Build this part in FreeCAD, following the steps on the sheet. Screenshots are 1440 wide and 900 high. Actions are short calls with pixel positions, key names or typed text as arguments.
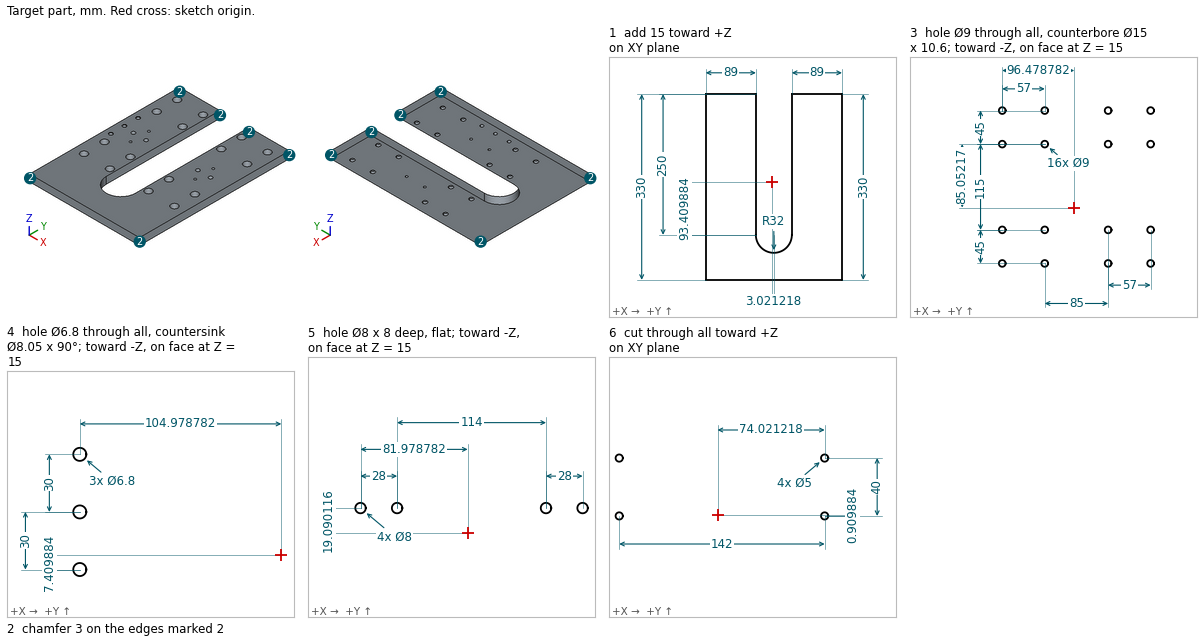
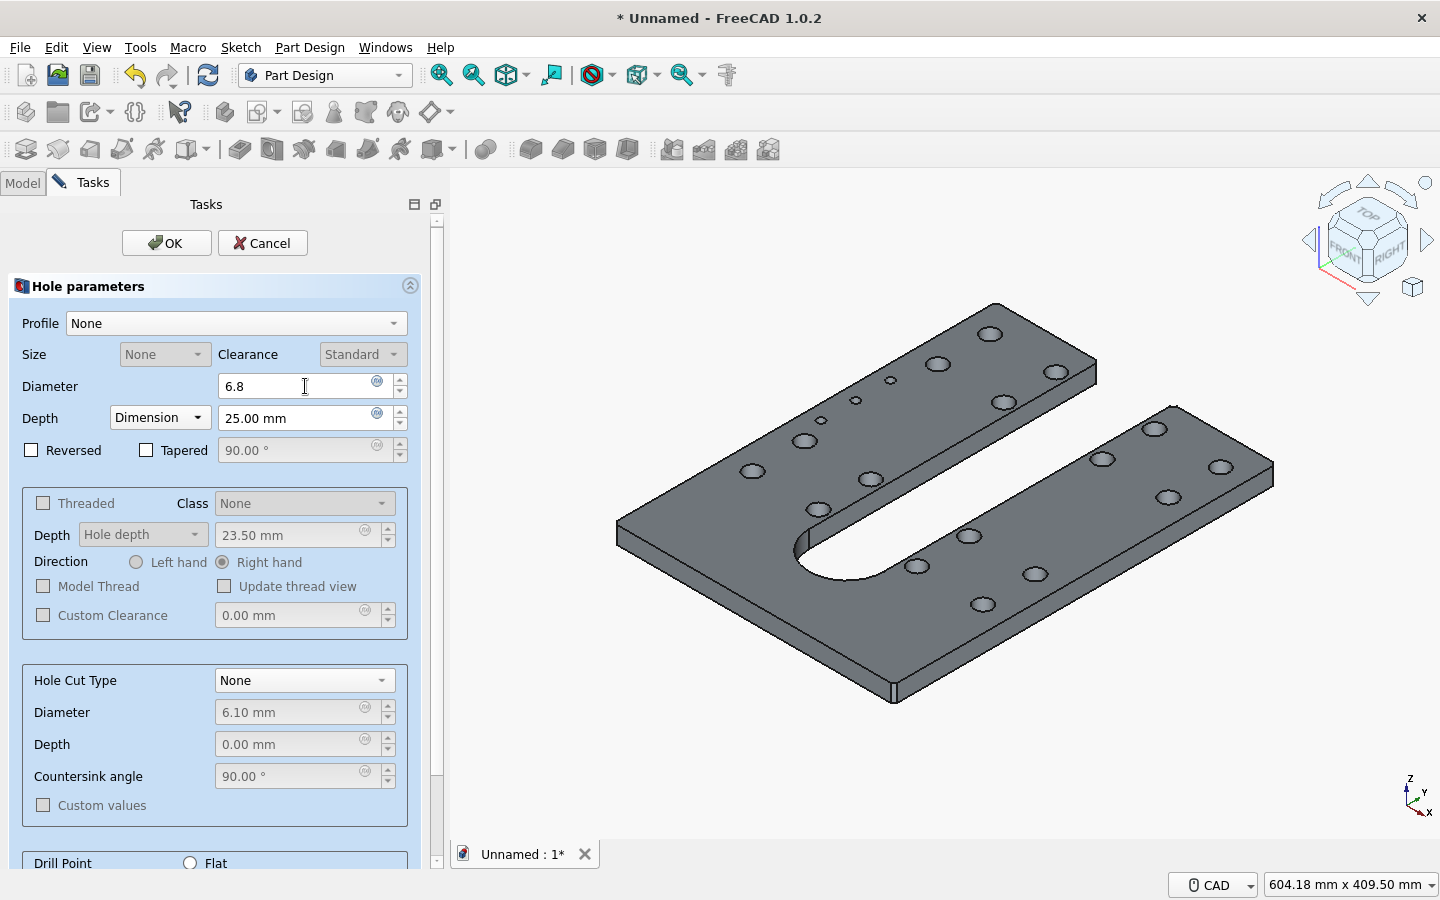
click(161, 418)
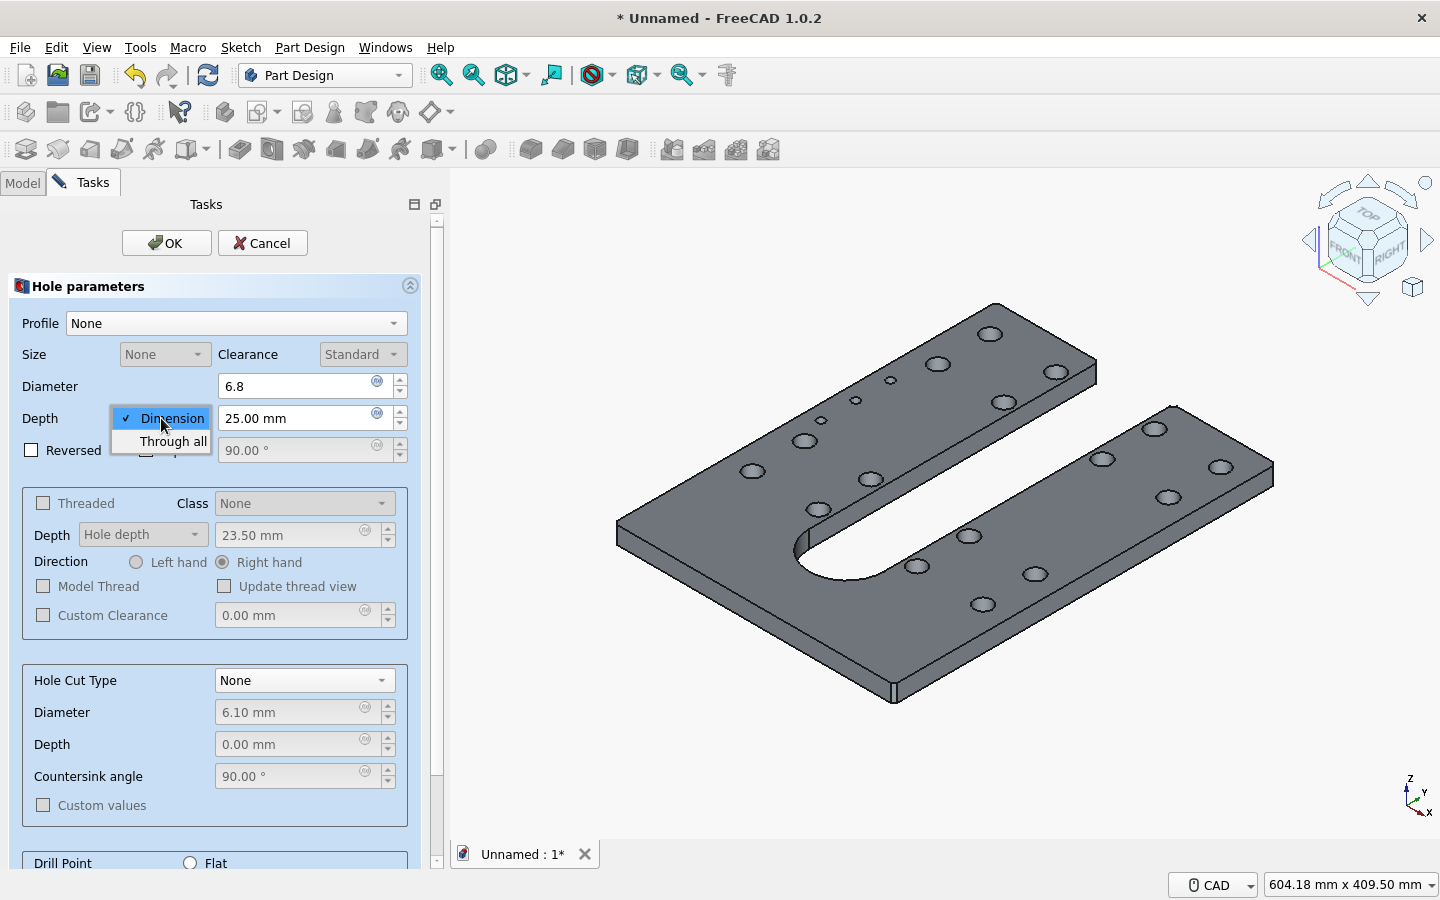
click(160, 442)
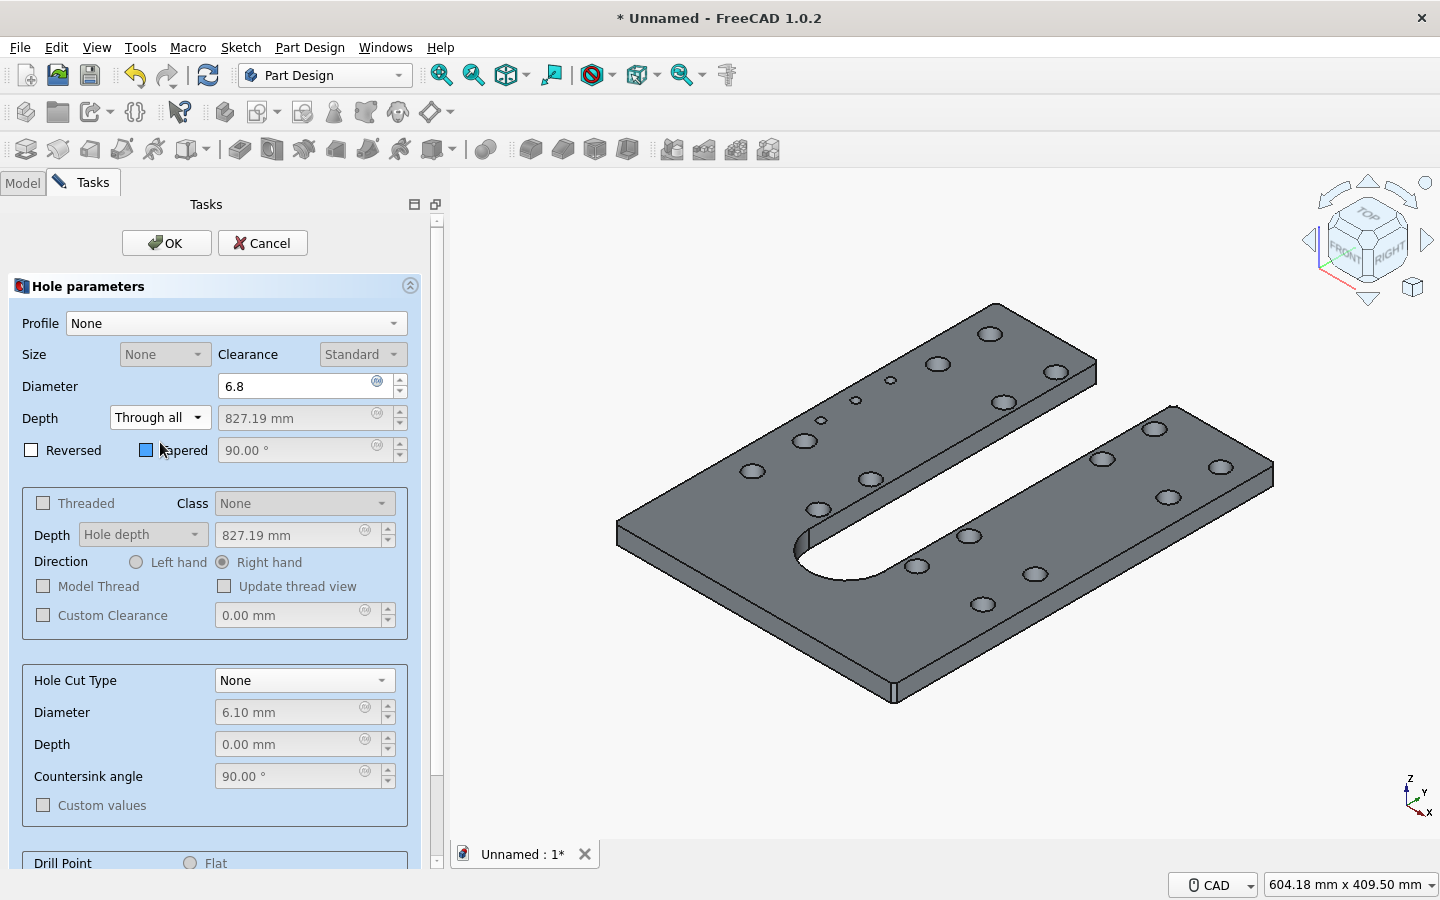
click(306, 680)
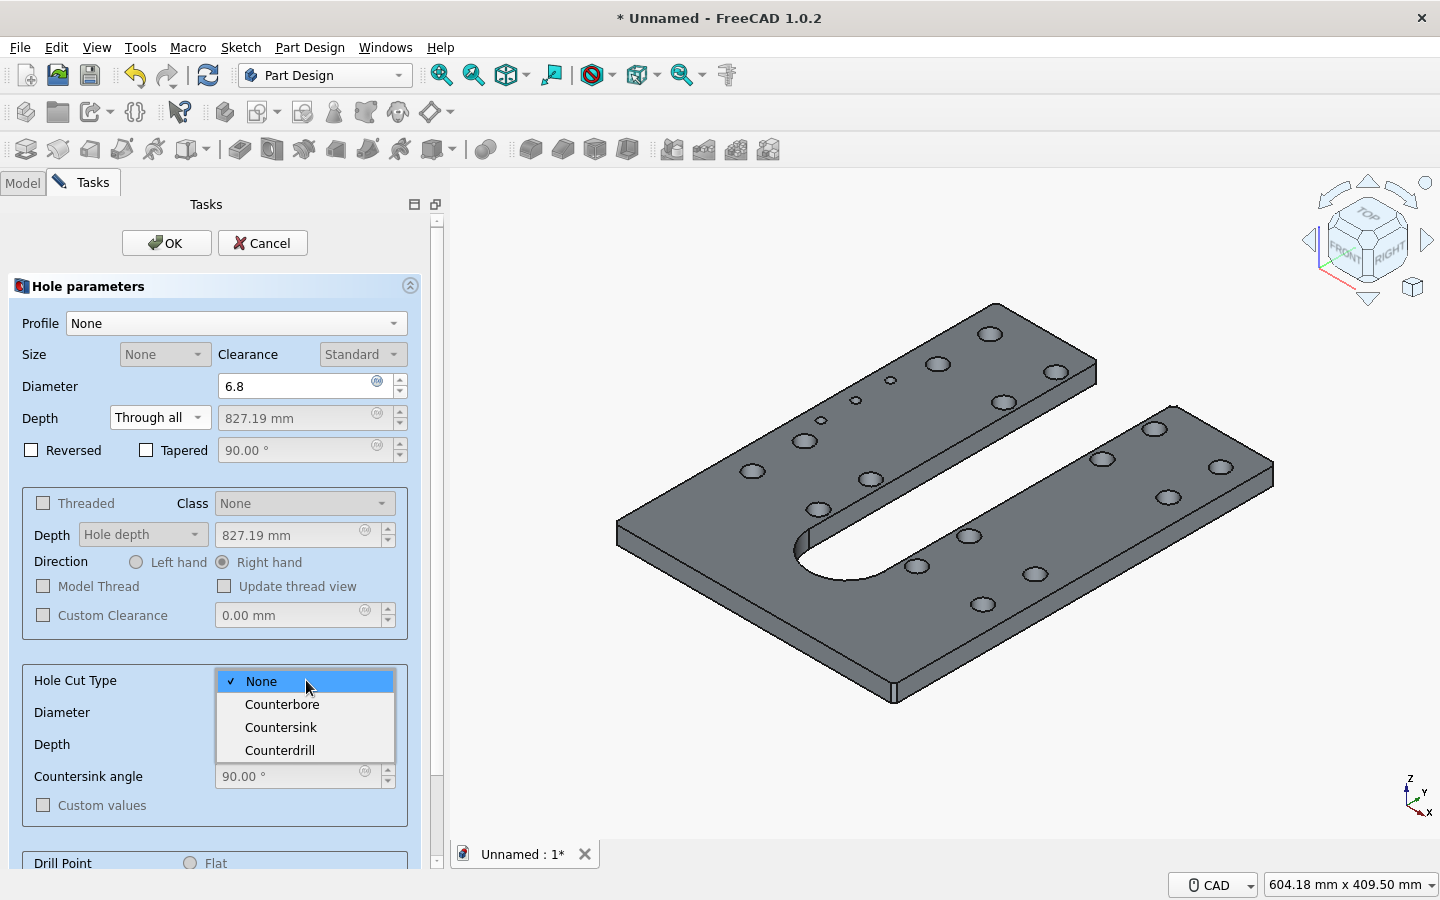
click(304, 728)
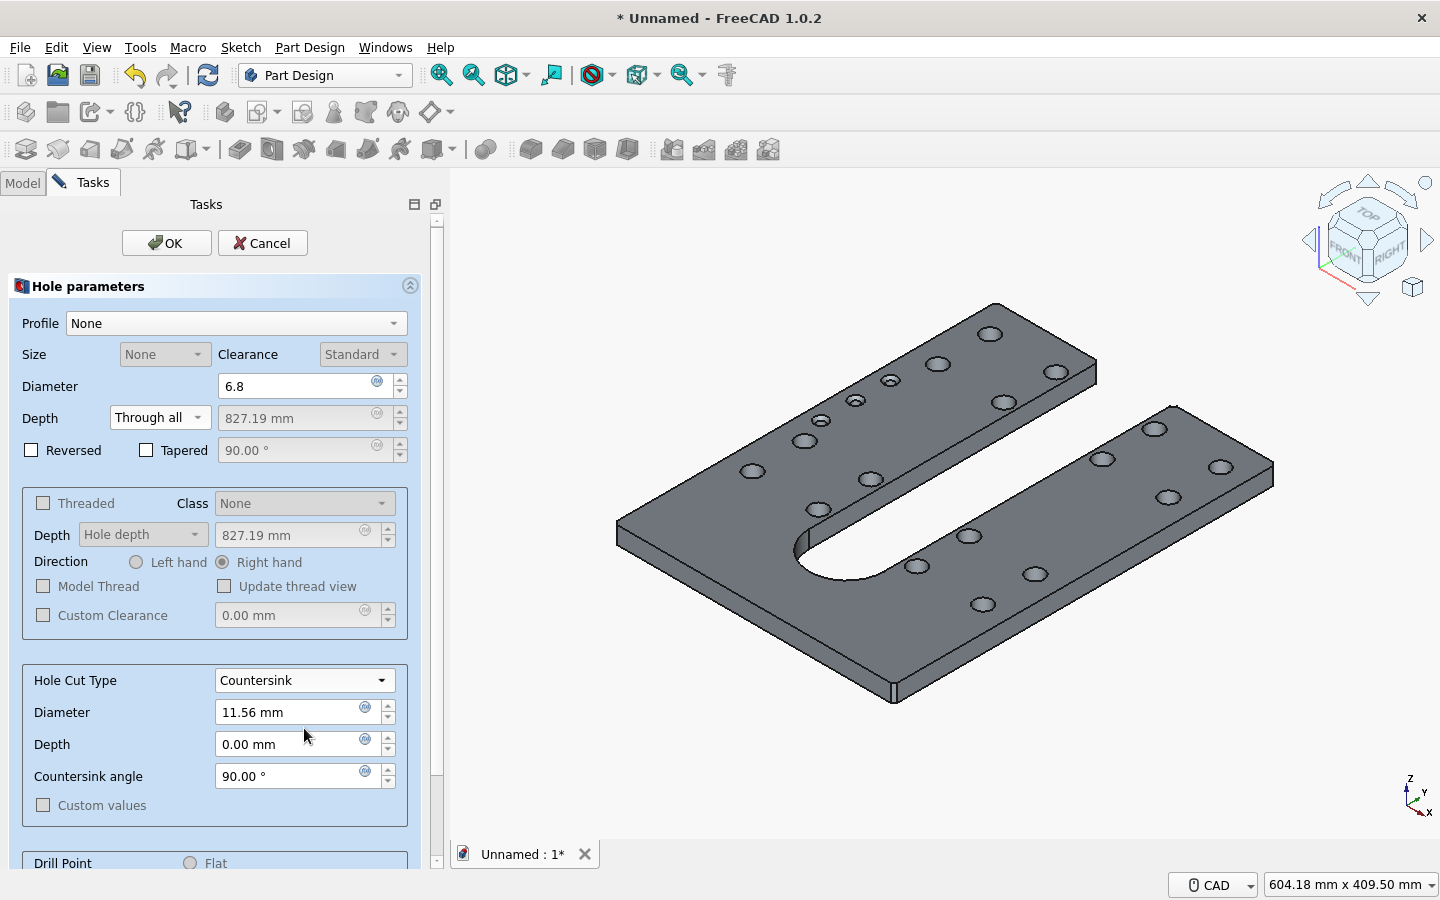
triple_click(298, 712)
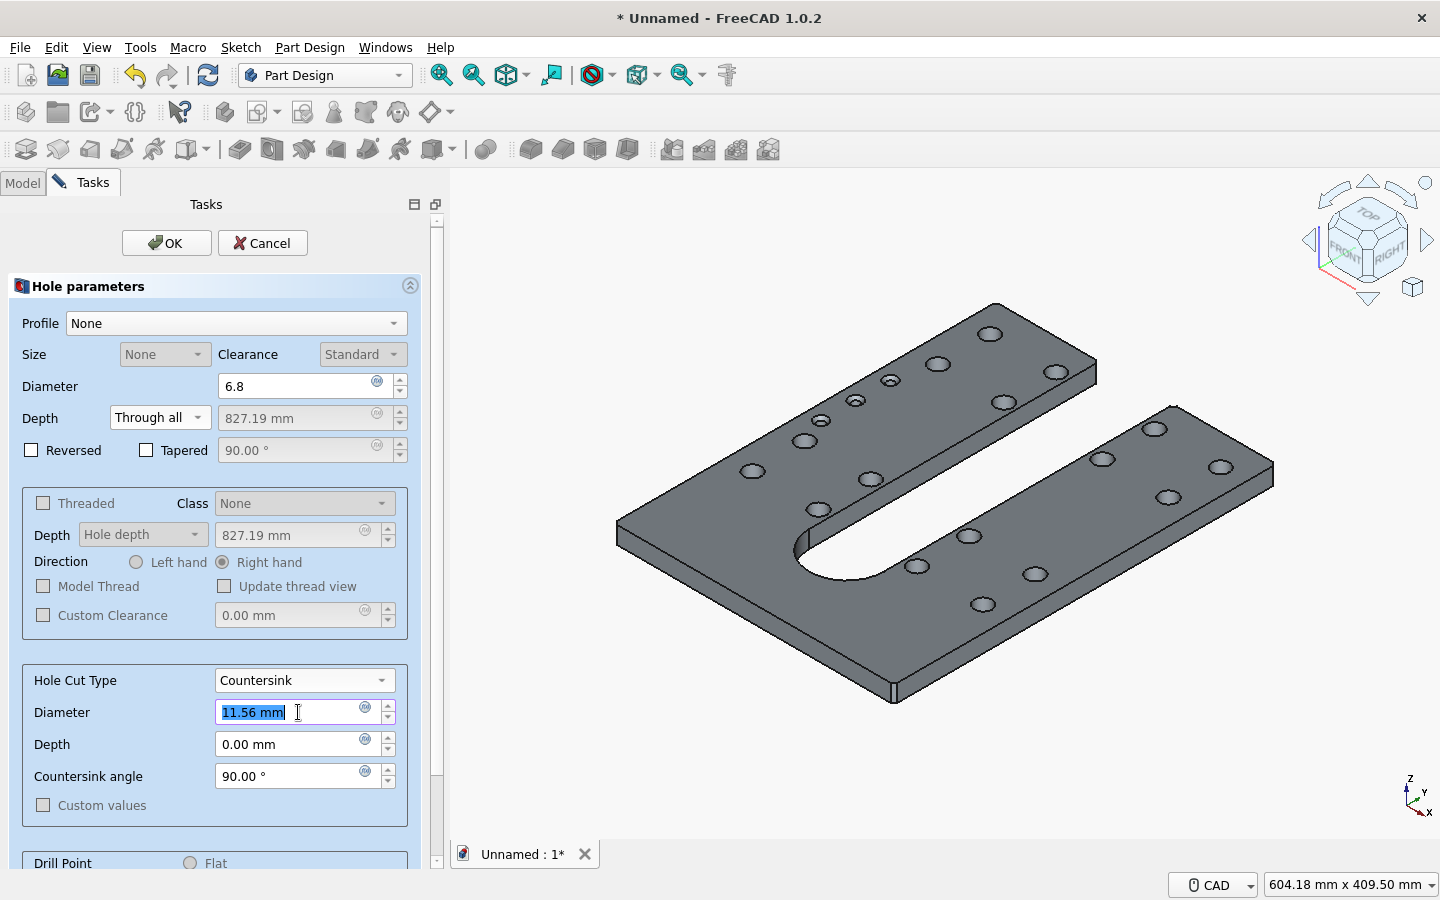
text(8.05)
key(Tab)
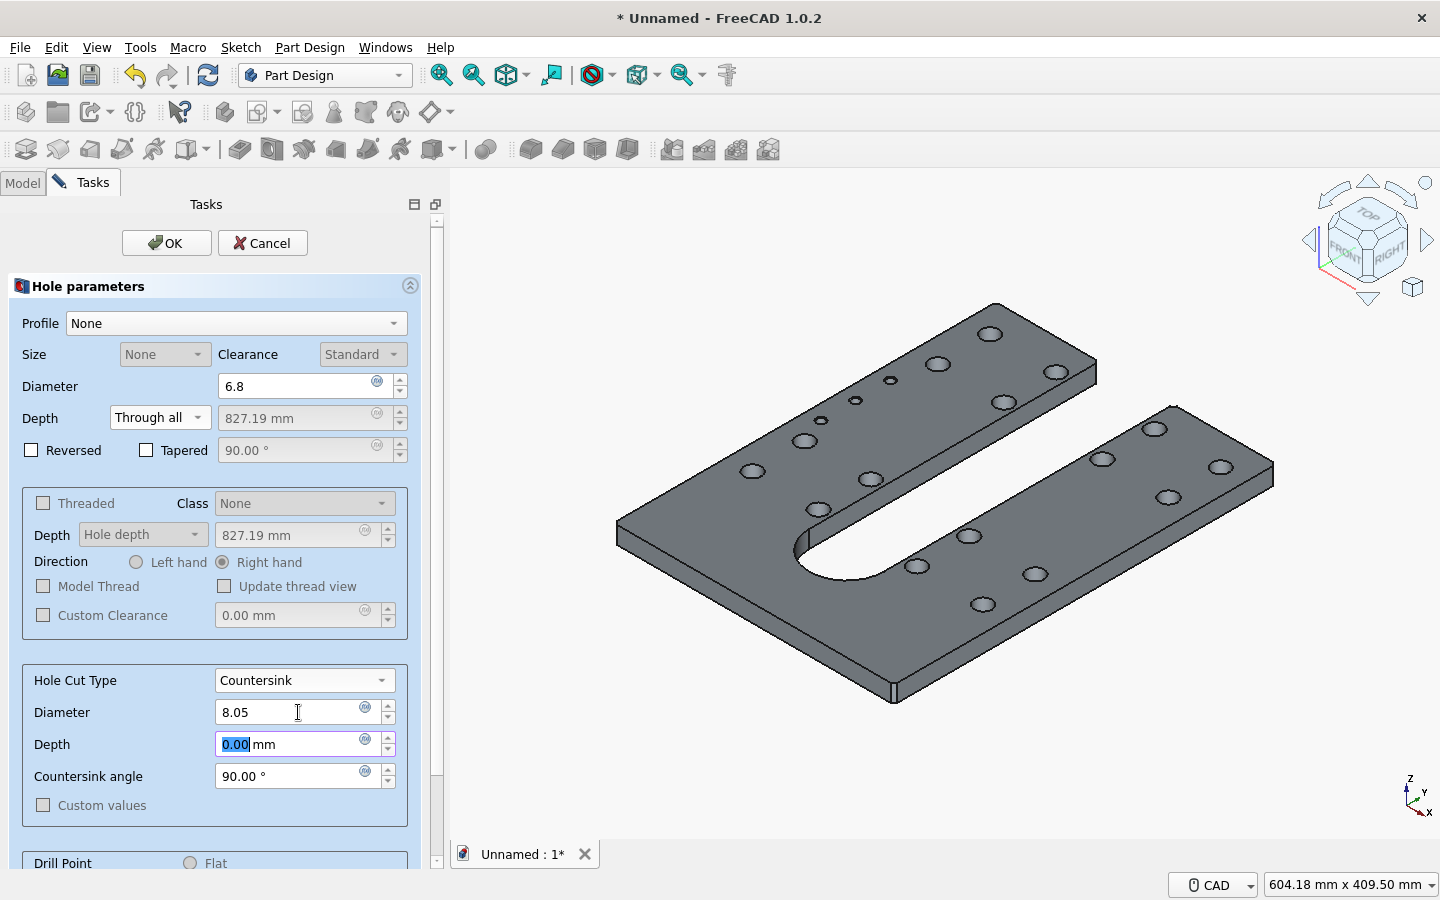
click(167, 243)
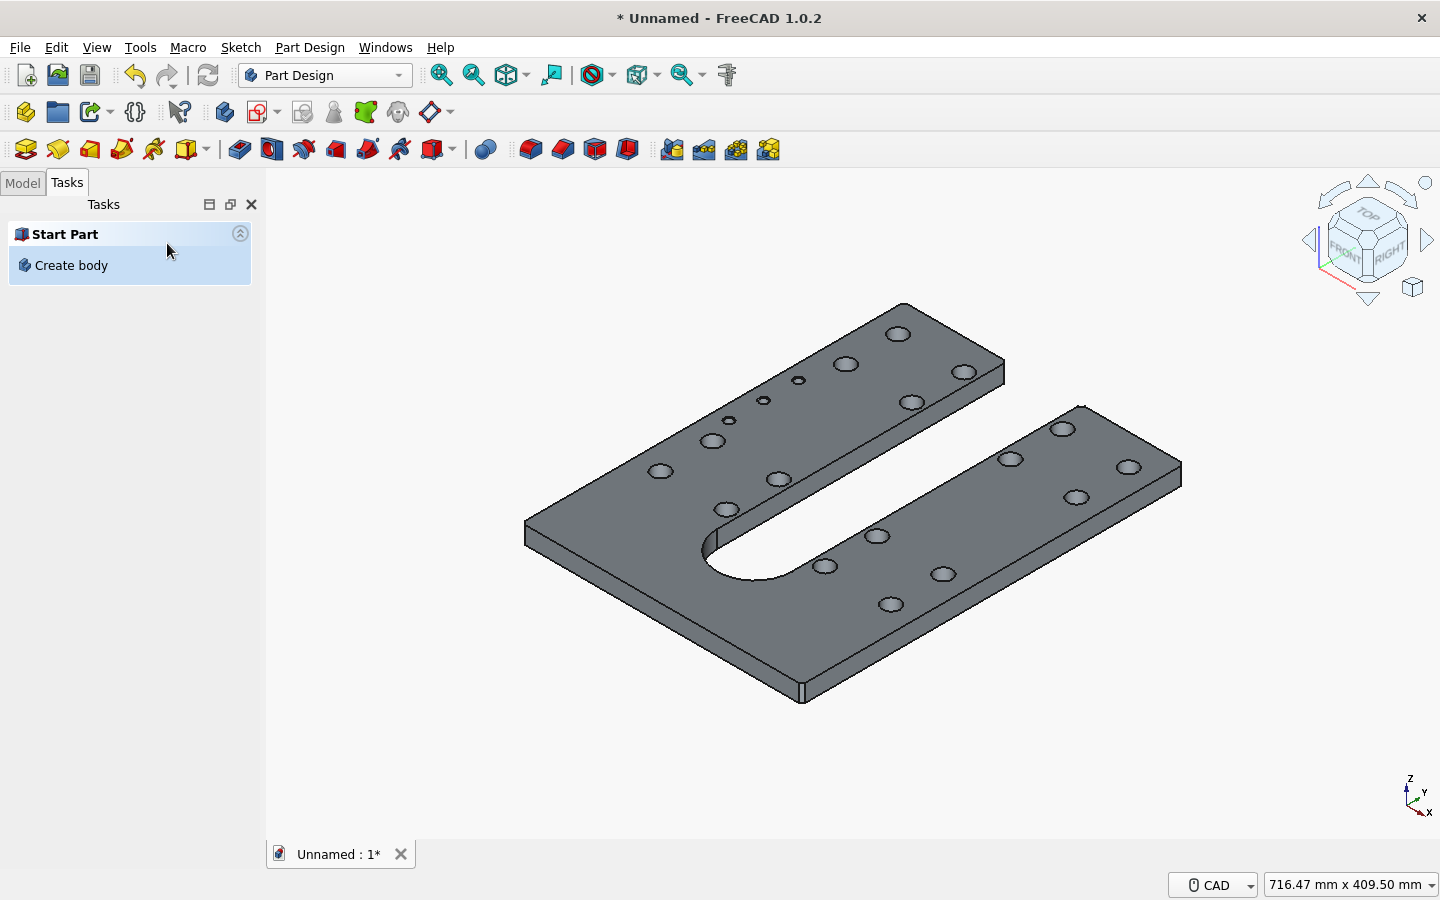
click(988, 507)